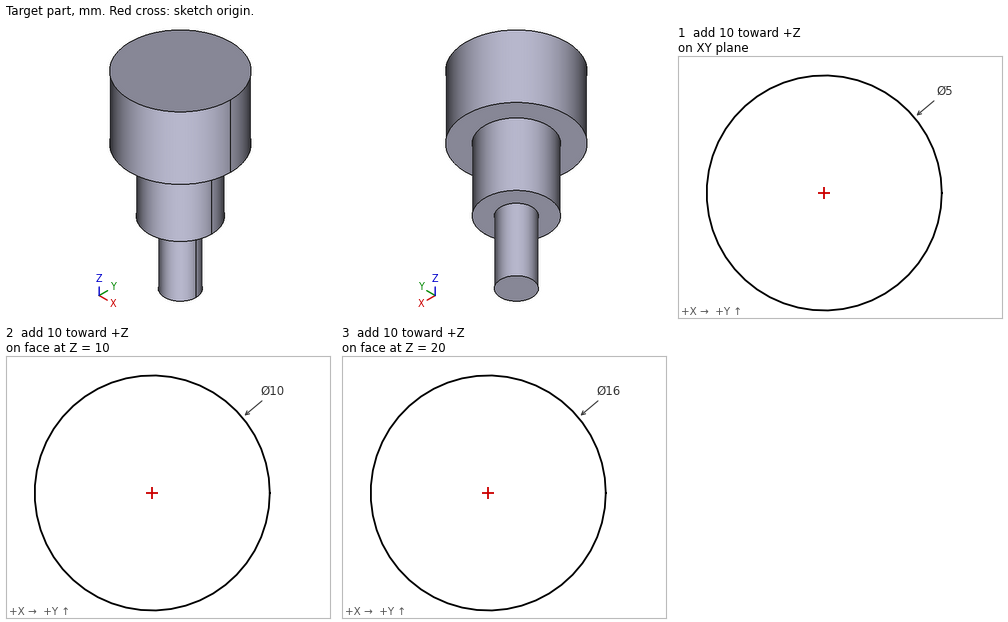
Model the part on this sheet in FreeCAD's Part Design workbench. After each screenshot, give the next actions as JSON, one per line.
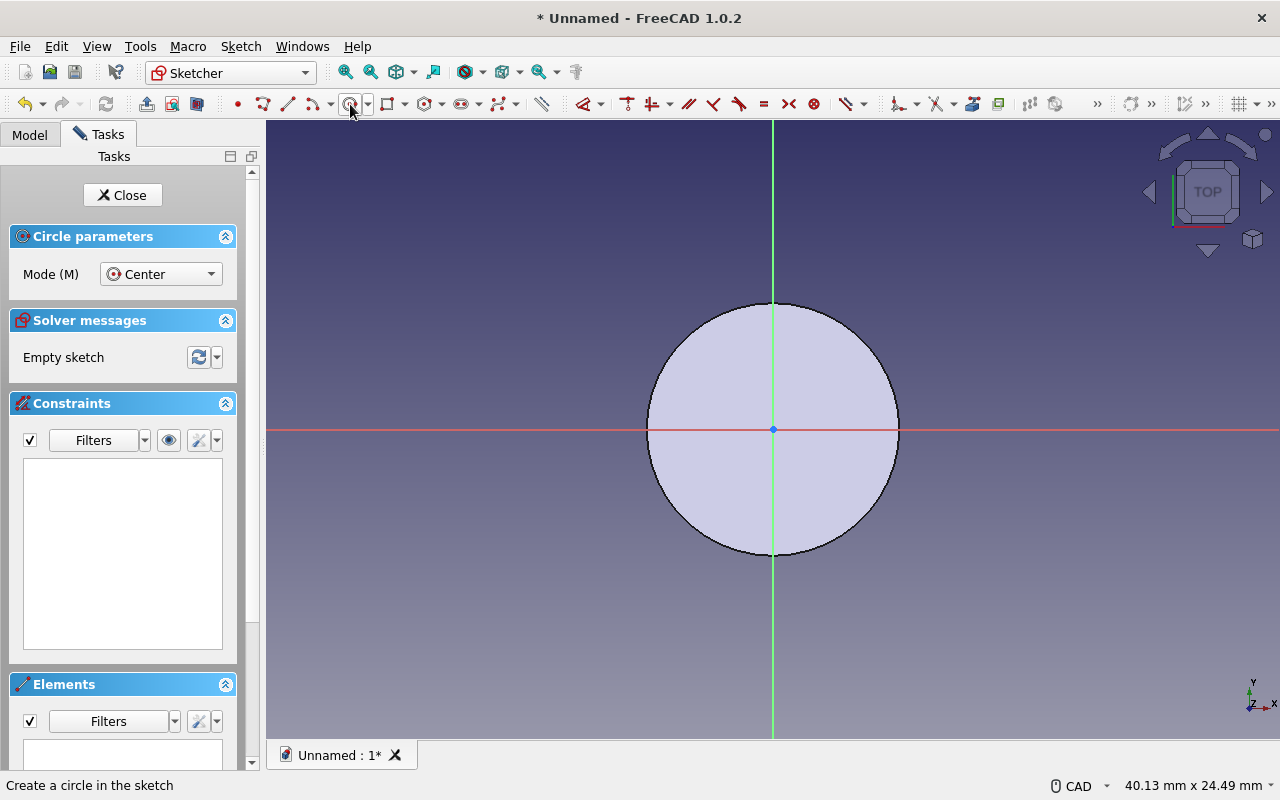
{"action": "left_click", "coordinate": [773, 430]}
{"action": "left_click", "coordinate": [916, 287]}
{"action": "key", "text": "Escape"}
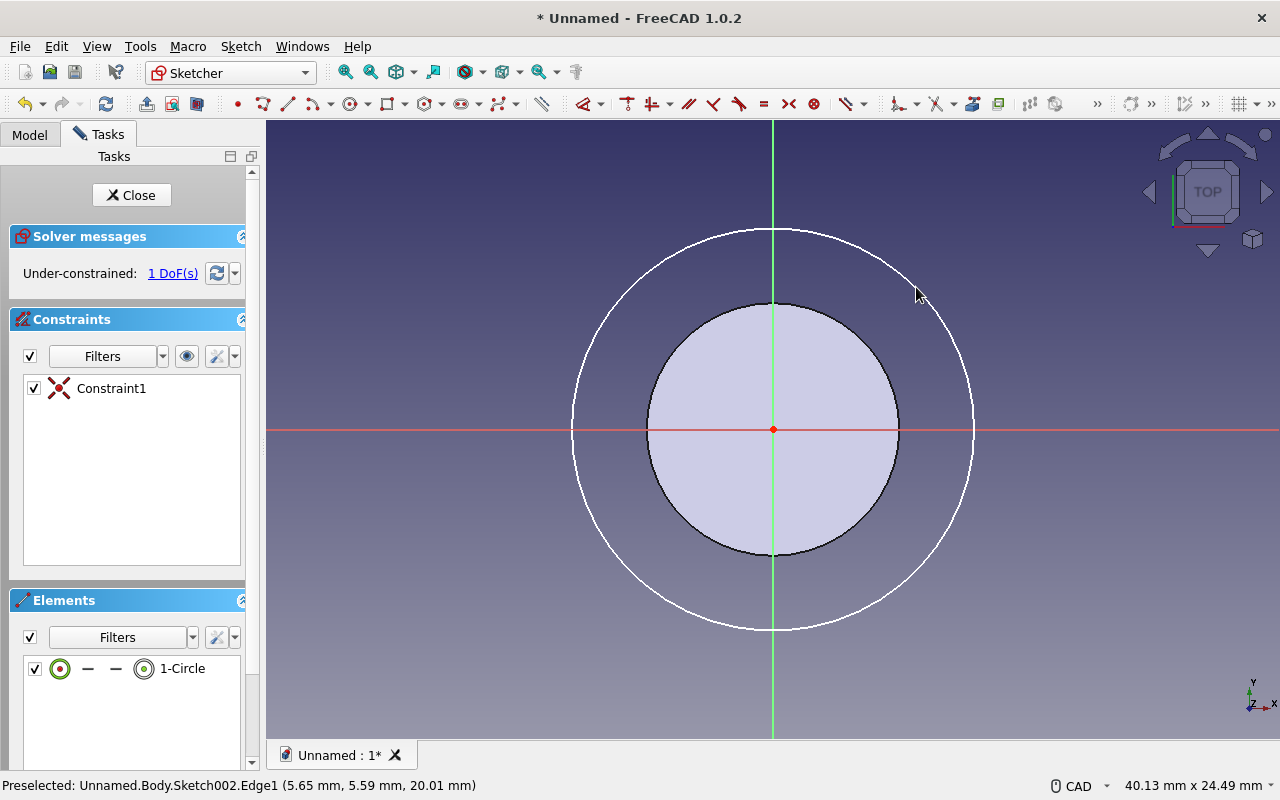
{"action": "key", "text": "d"}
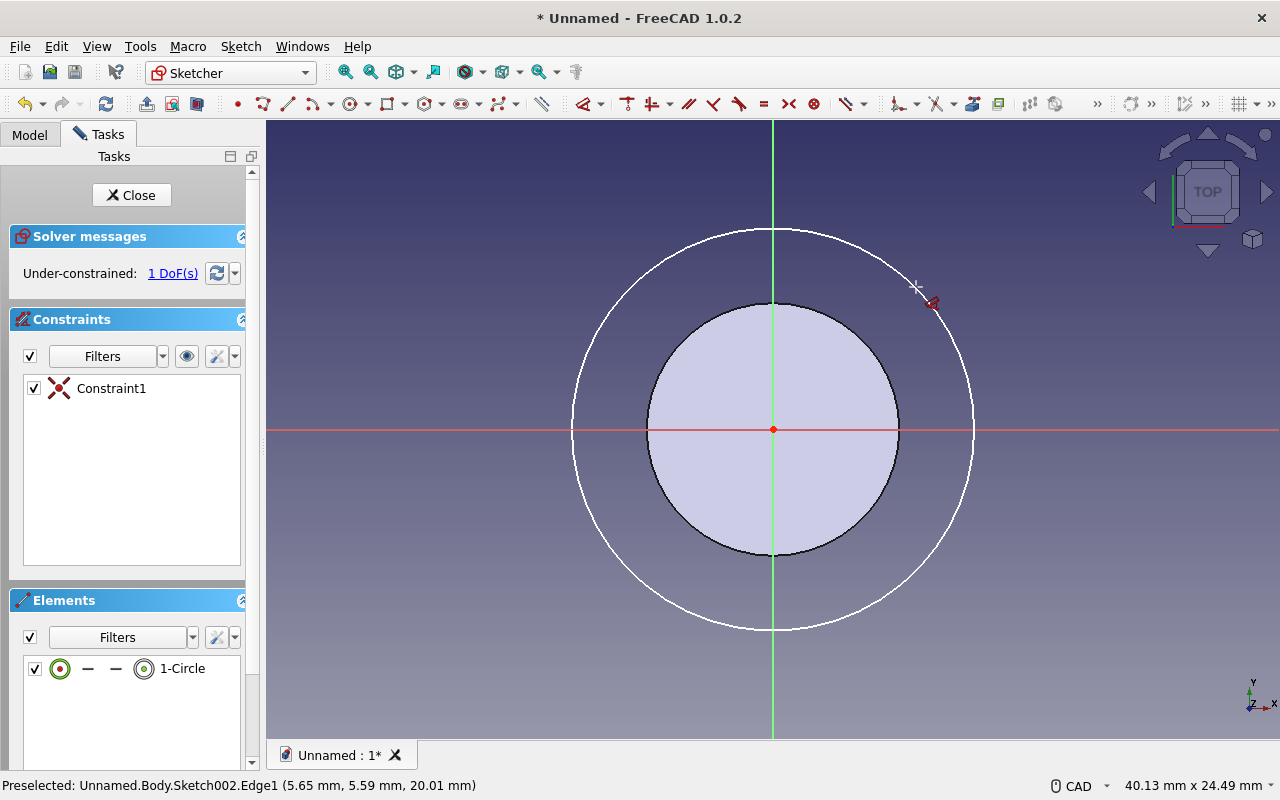
{"action": "left_click", "coordinate": [915, 287]}
{"action": "left_click", "coordinate": [938, 264]}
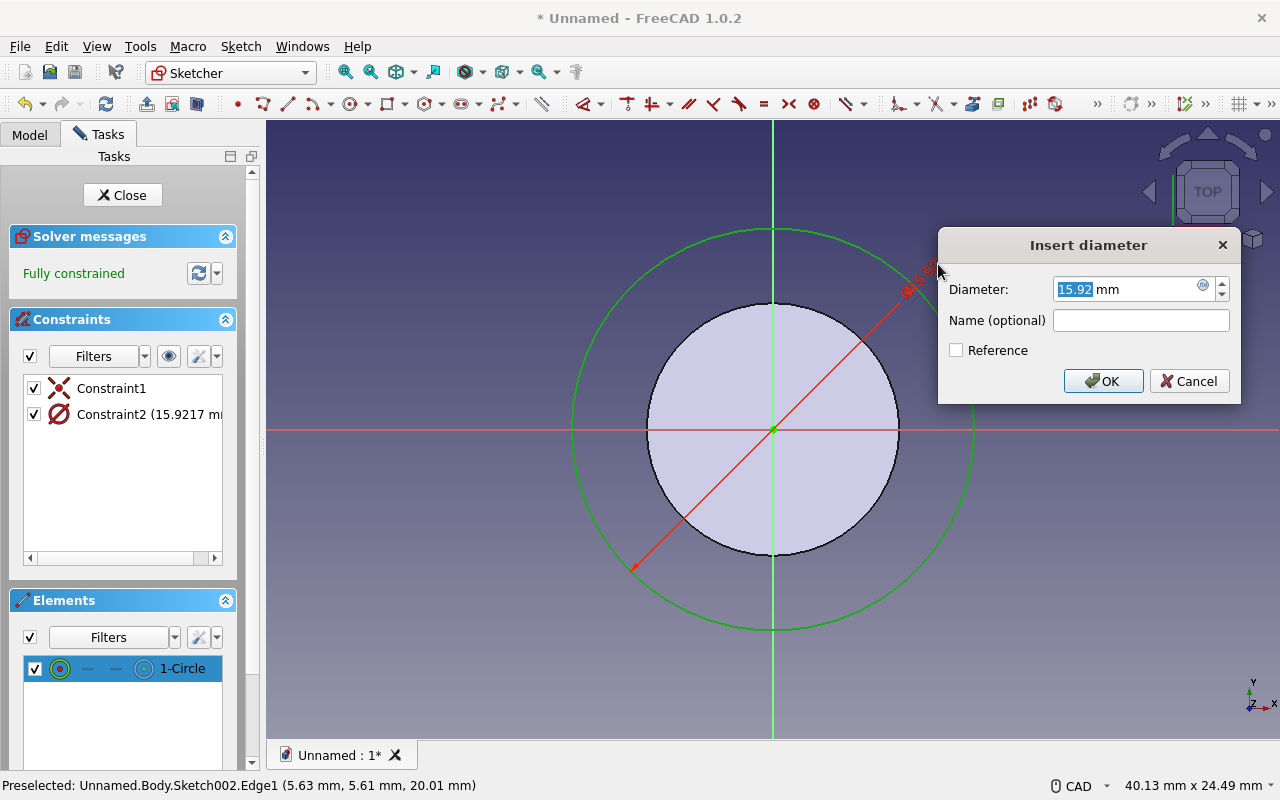
{"action": "type", "text": "16"}
{"action": "key", "text": "Return"}
{"action": "key", "text": "Escape"}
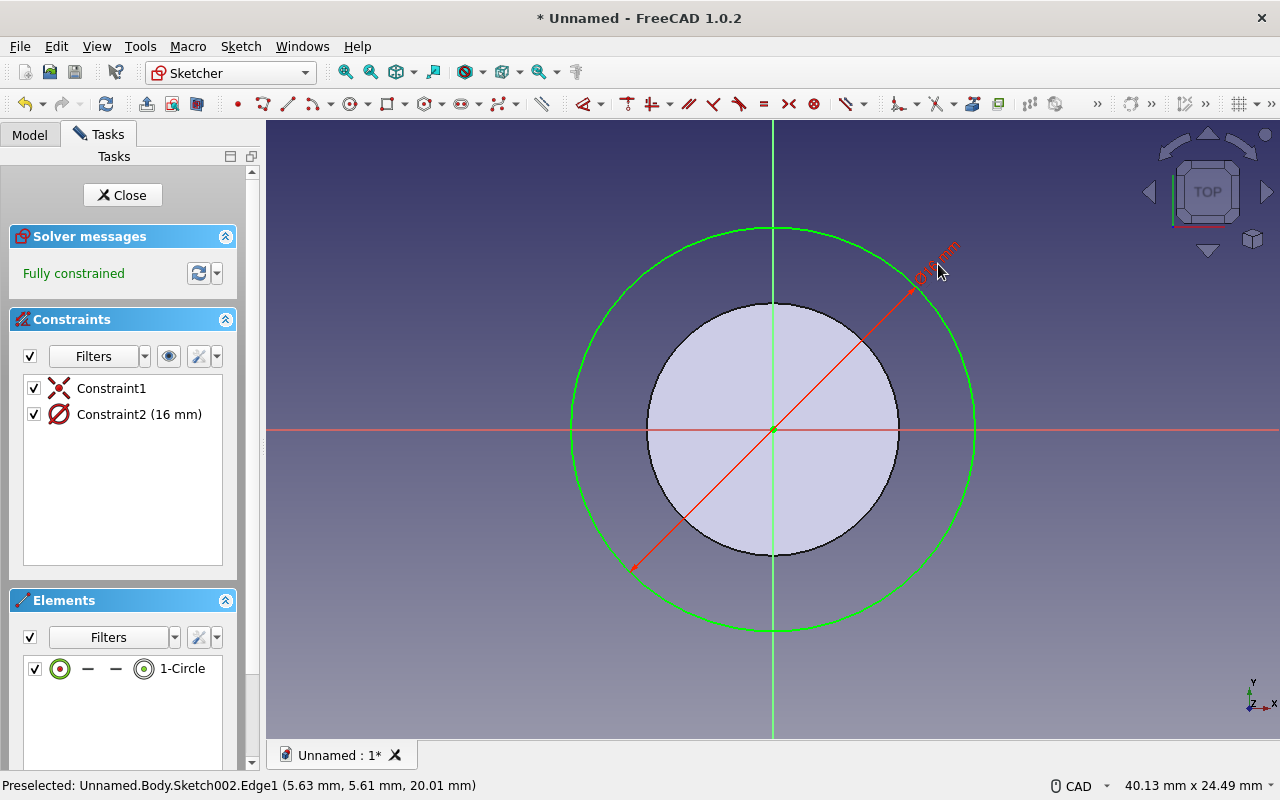
{"action": "left_click", "coordinate": [123, 195]}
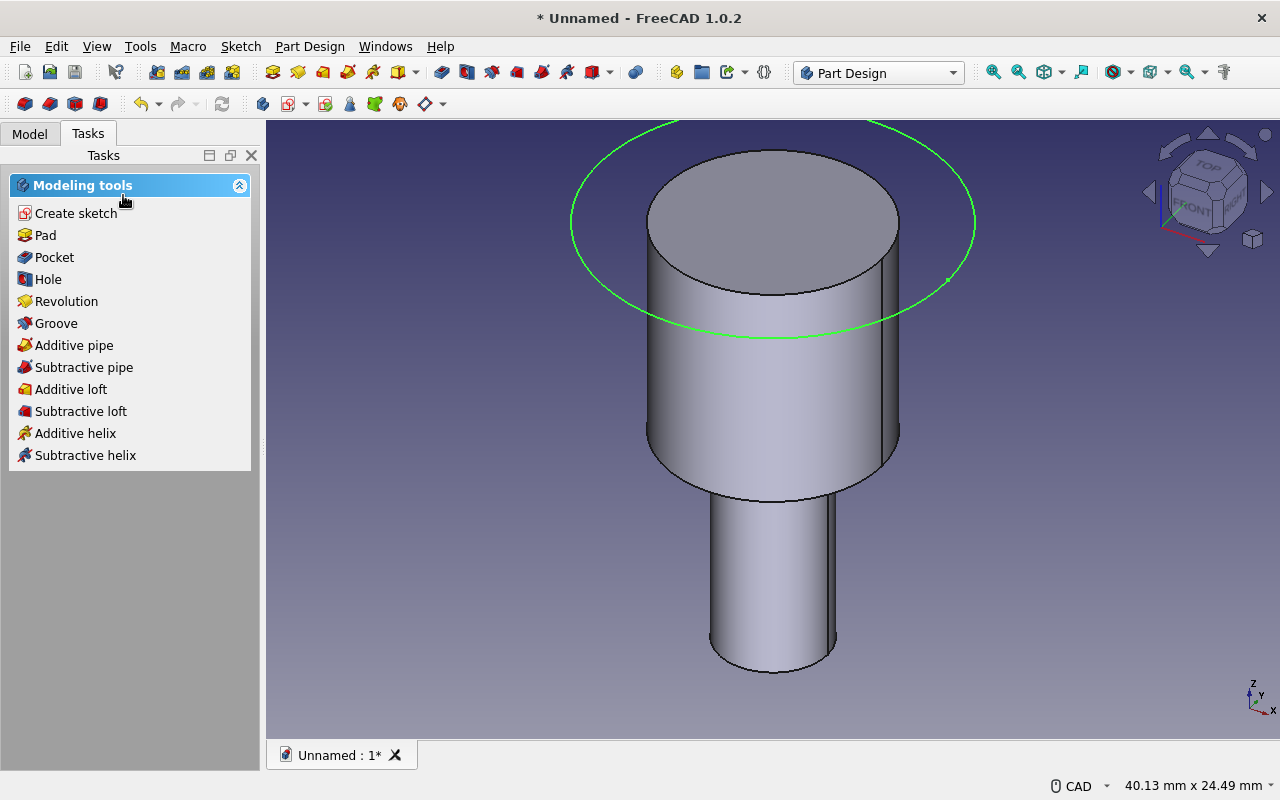
{"action": "left_click", "coordinate": [273, 72]}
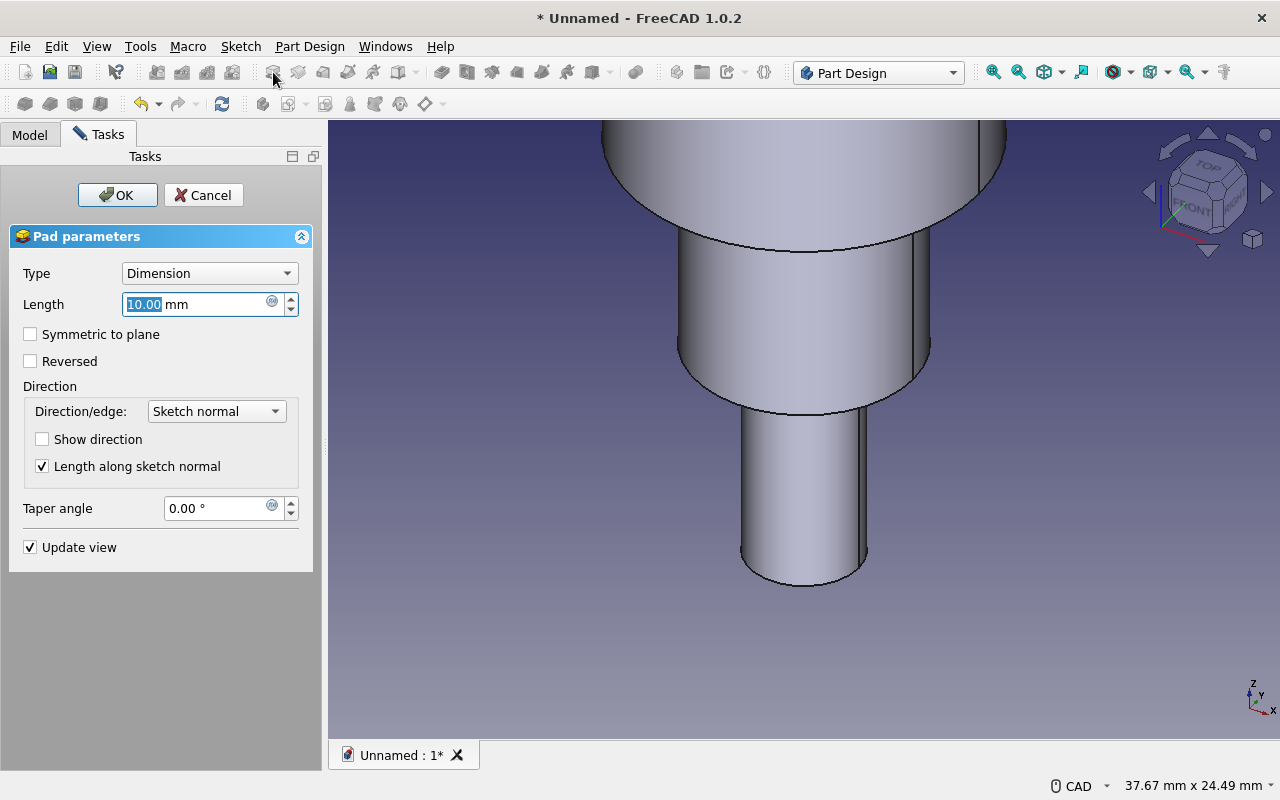
{"action": "type", "text": "10"}
{"action": "key", "text": "Tab"}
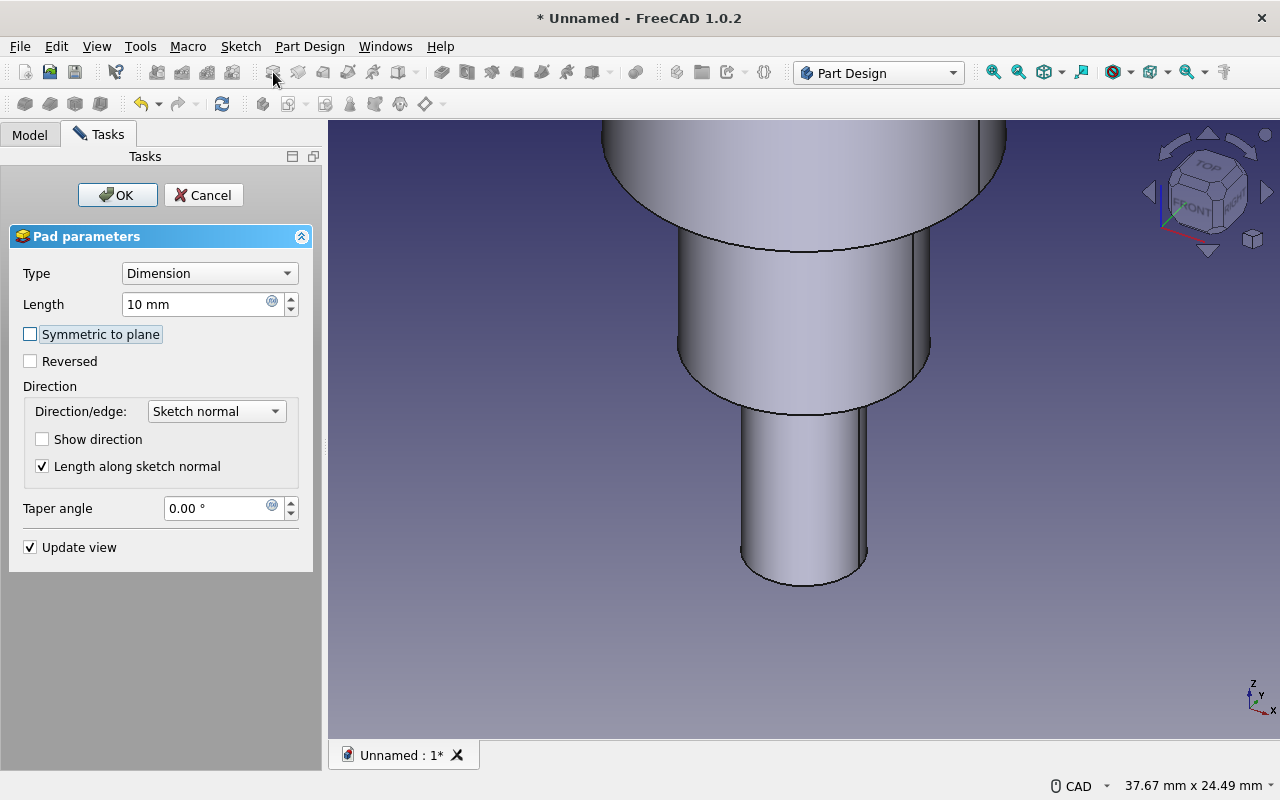
{"action": "left_click", "coordinate": [118, 195]}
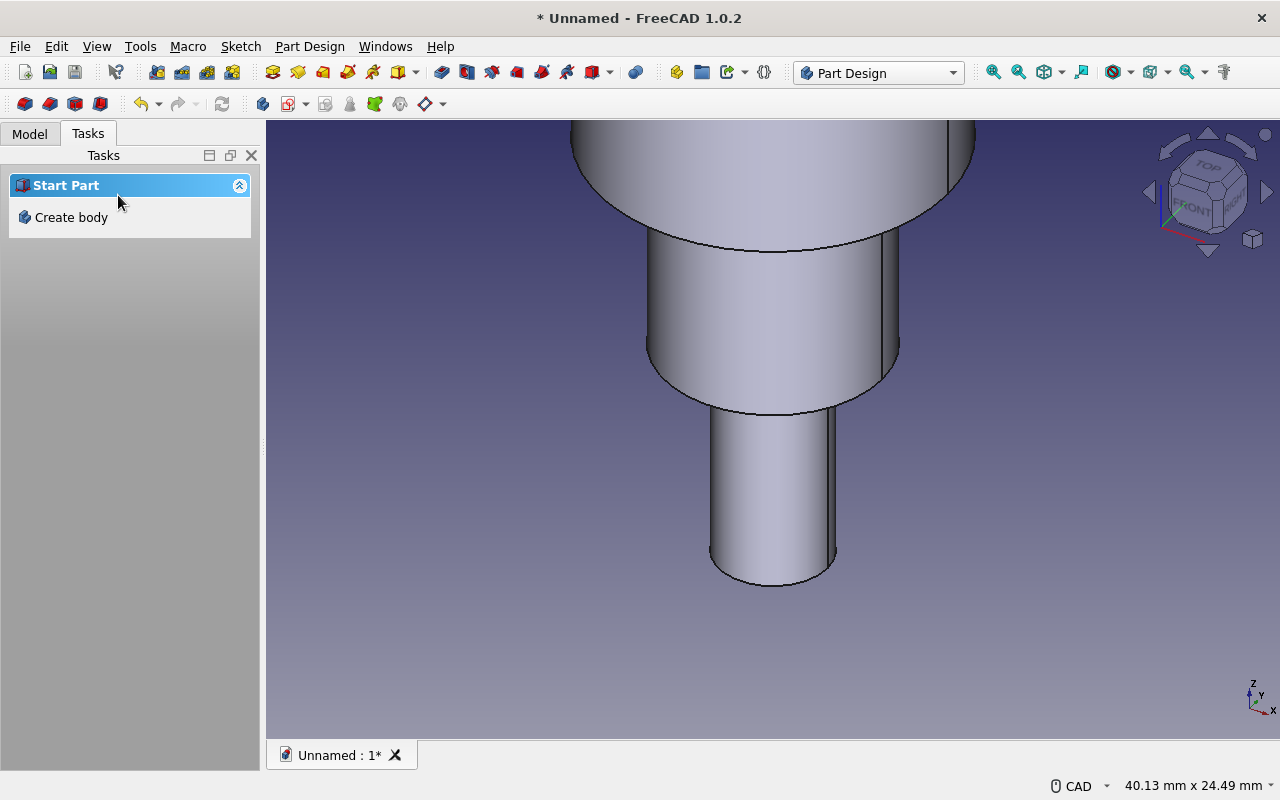
{"action": "key", "text": "0"}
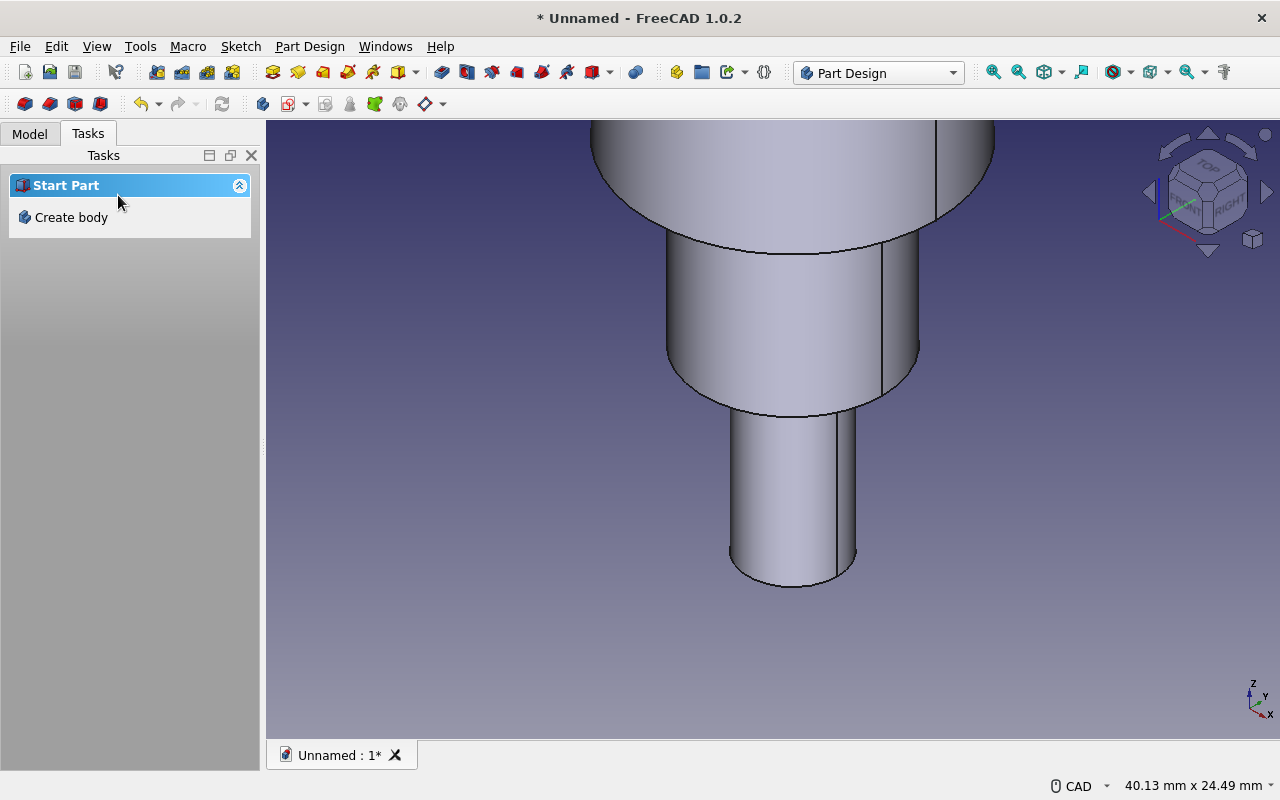
{"action": "left_click", "coordinate": [994, 72]}